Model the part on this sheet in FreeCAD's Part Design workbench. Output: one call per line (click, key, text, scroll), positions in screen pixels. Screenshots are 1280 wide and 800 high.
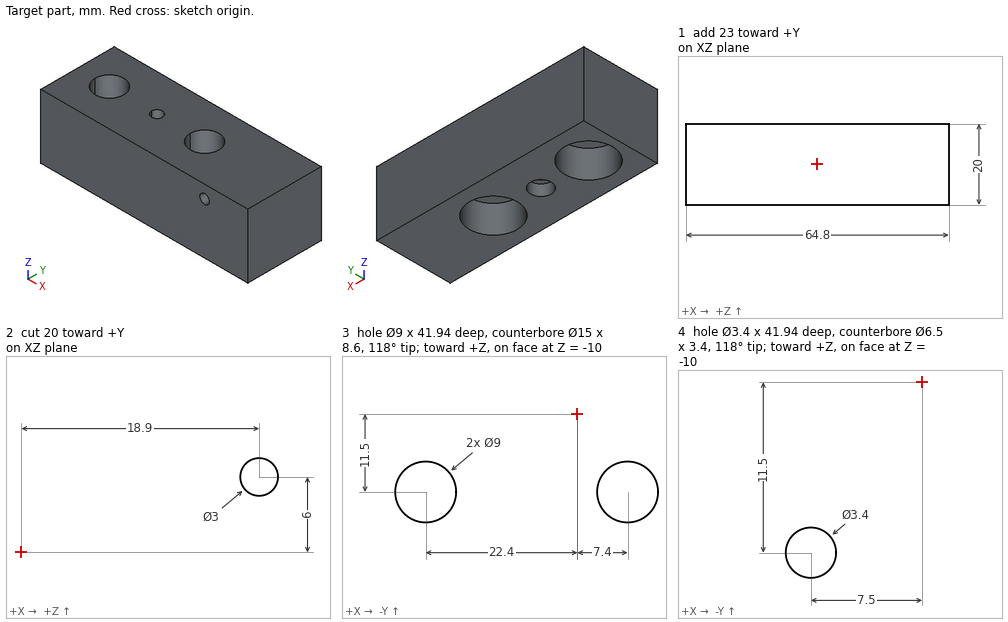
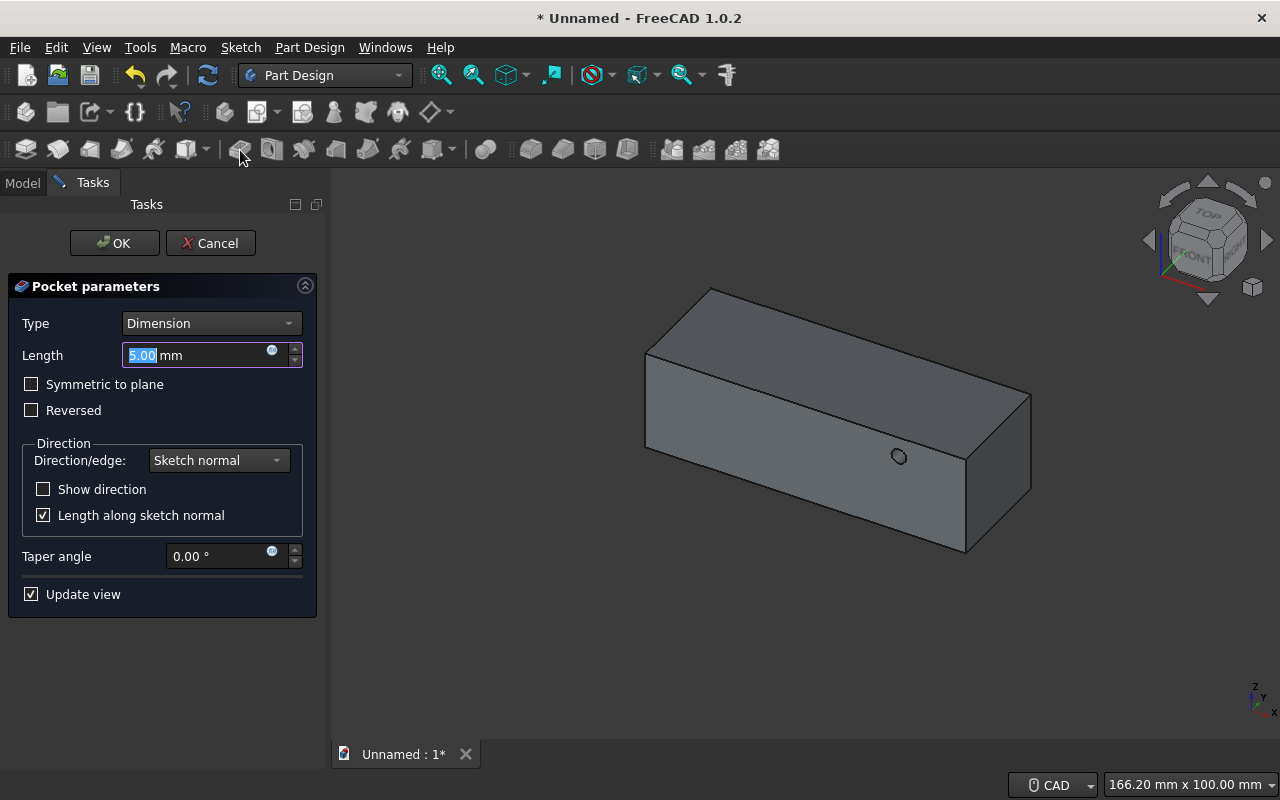
text(20)
key(Tab)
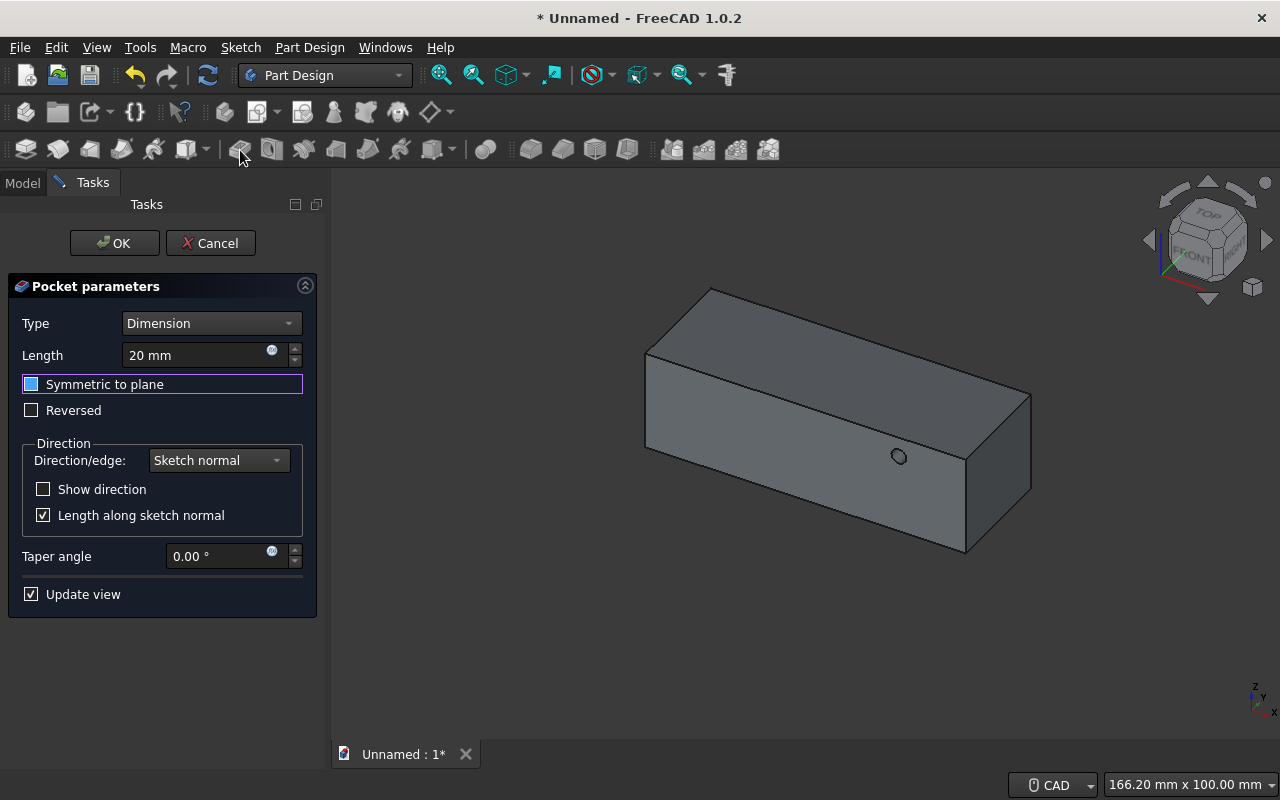
click(115, 243)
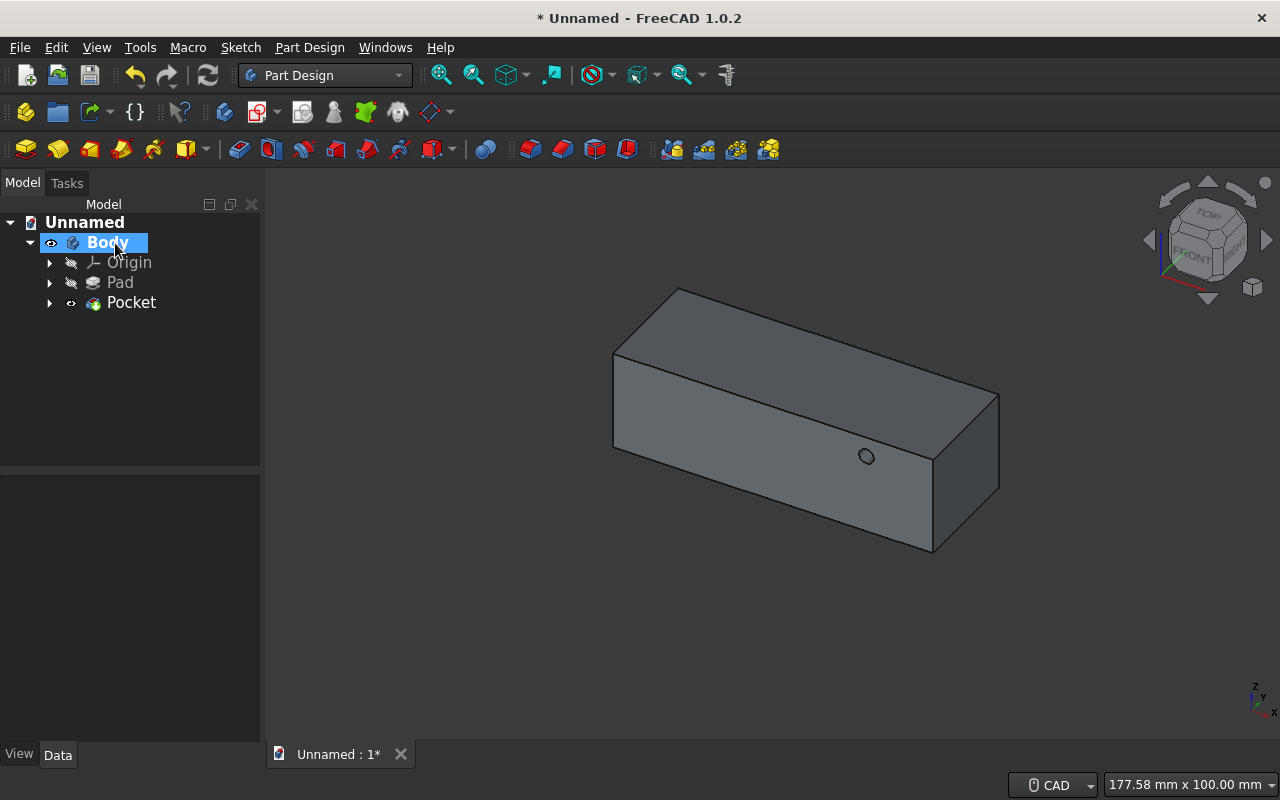
key(5)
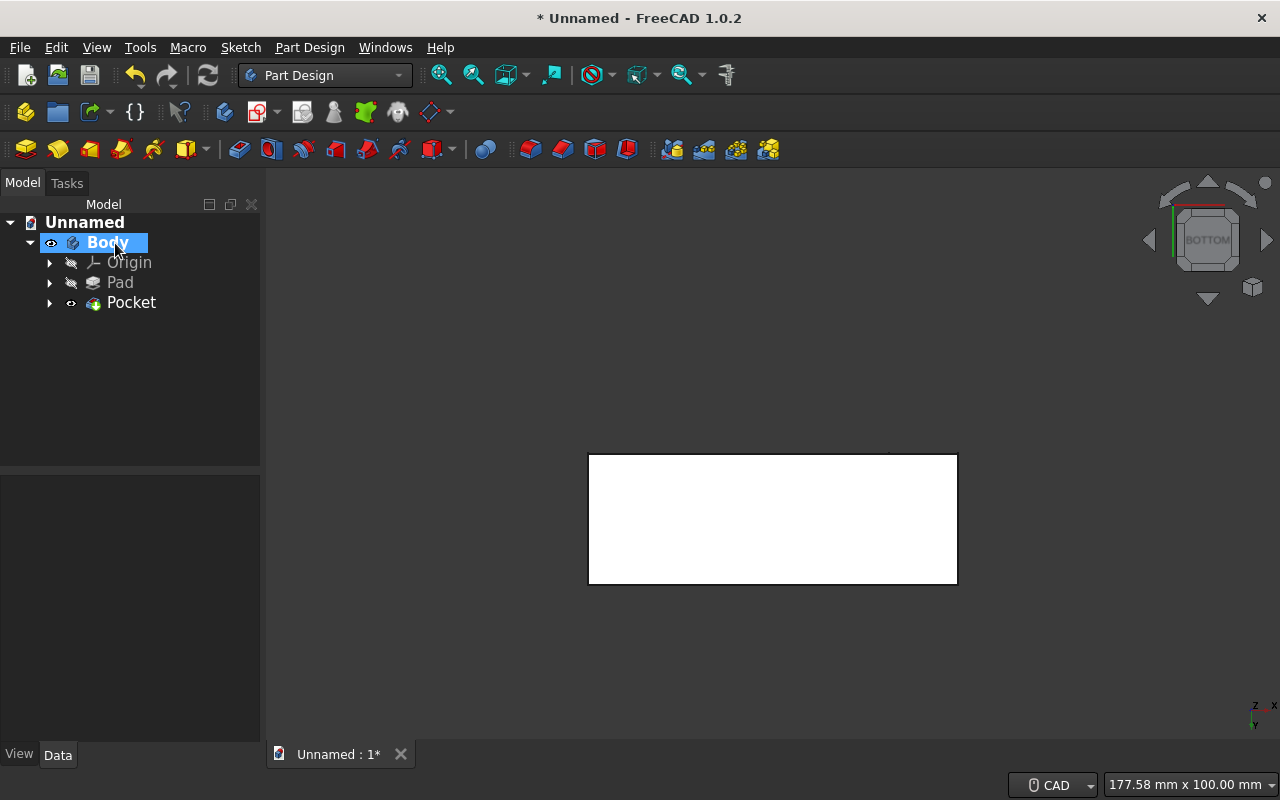
click(442, 76)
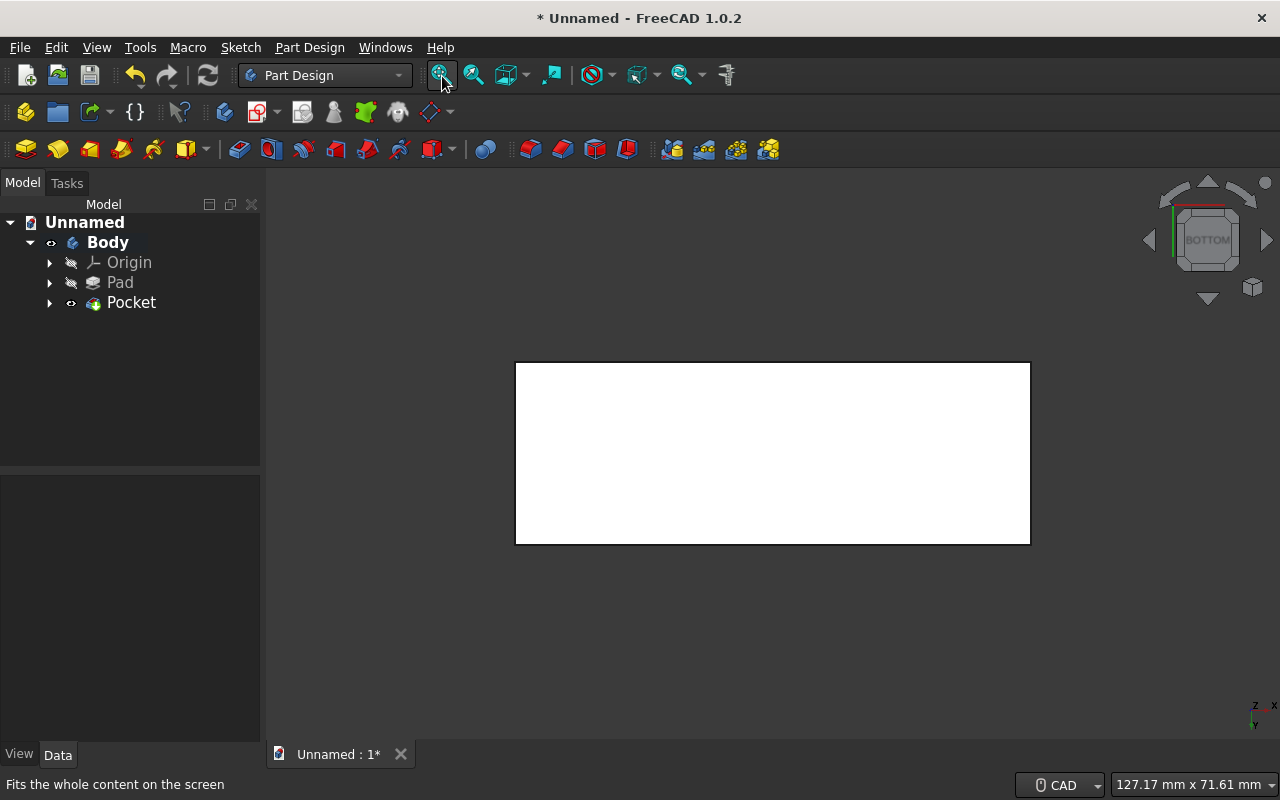
click(921, 452)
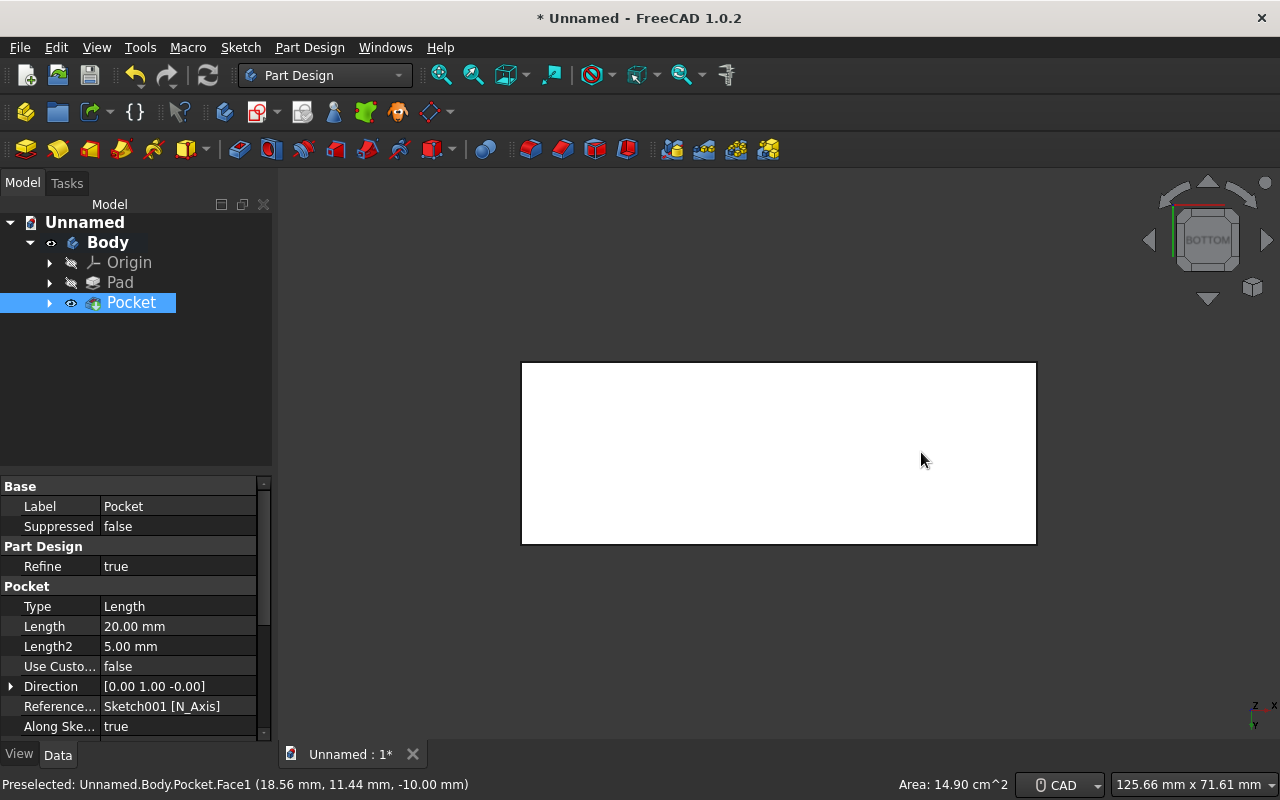
click(258, 112)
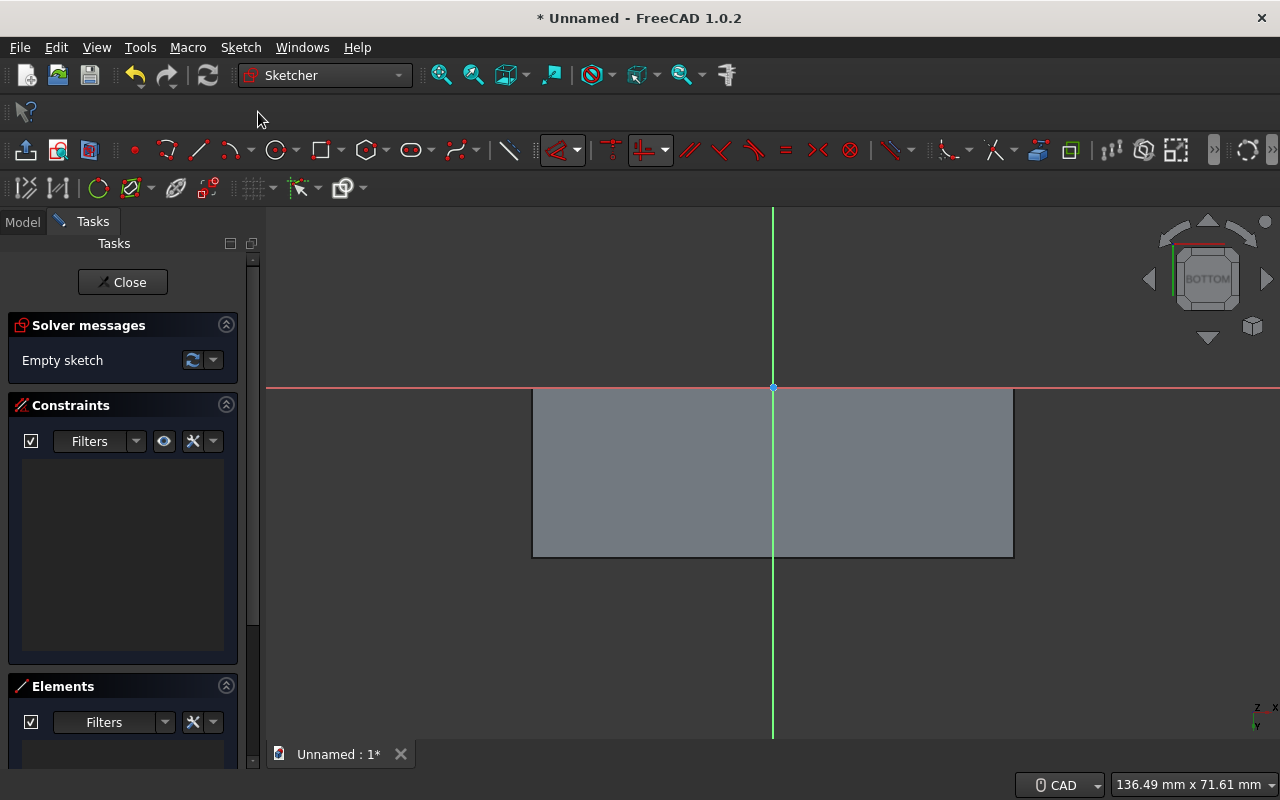
scroll(733, 415, up, 3)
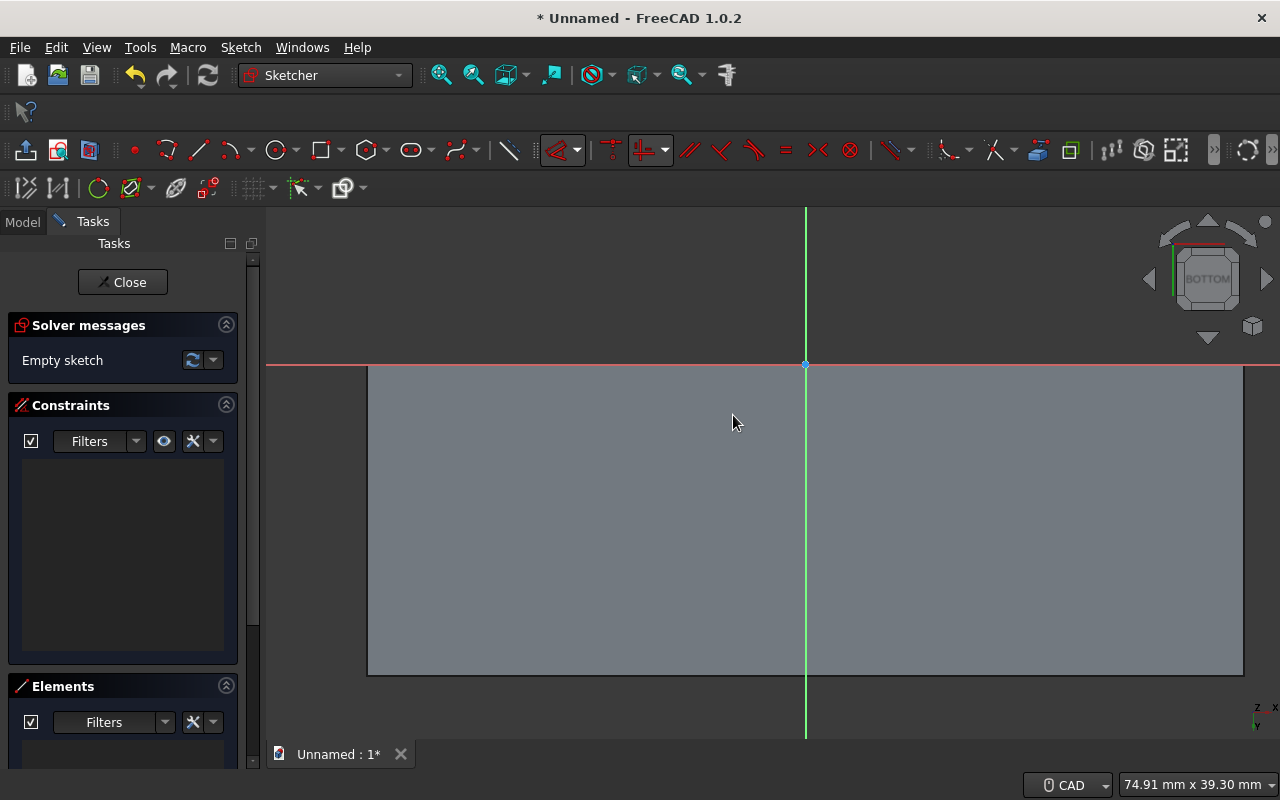
click(276, 150)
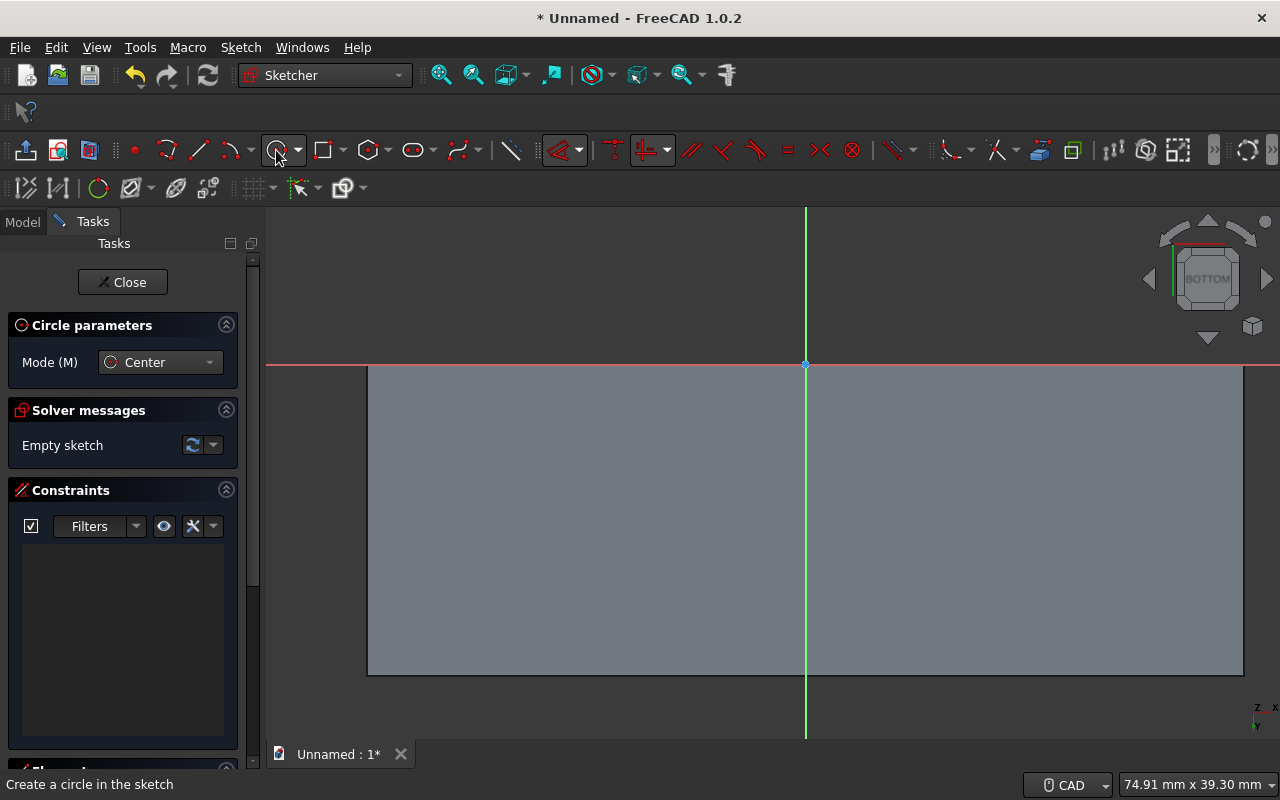
click(502, 520)
move(545, 477)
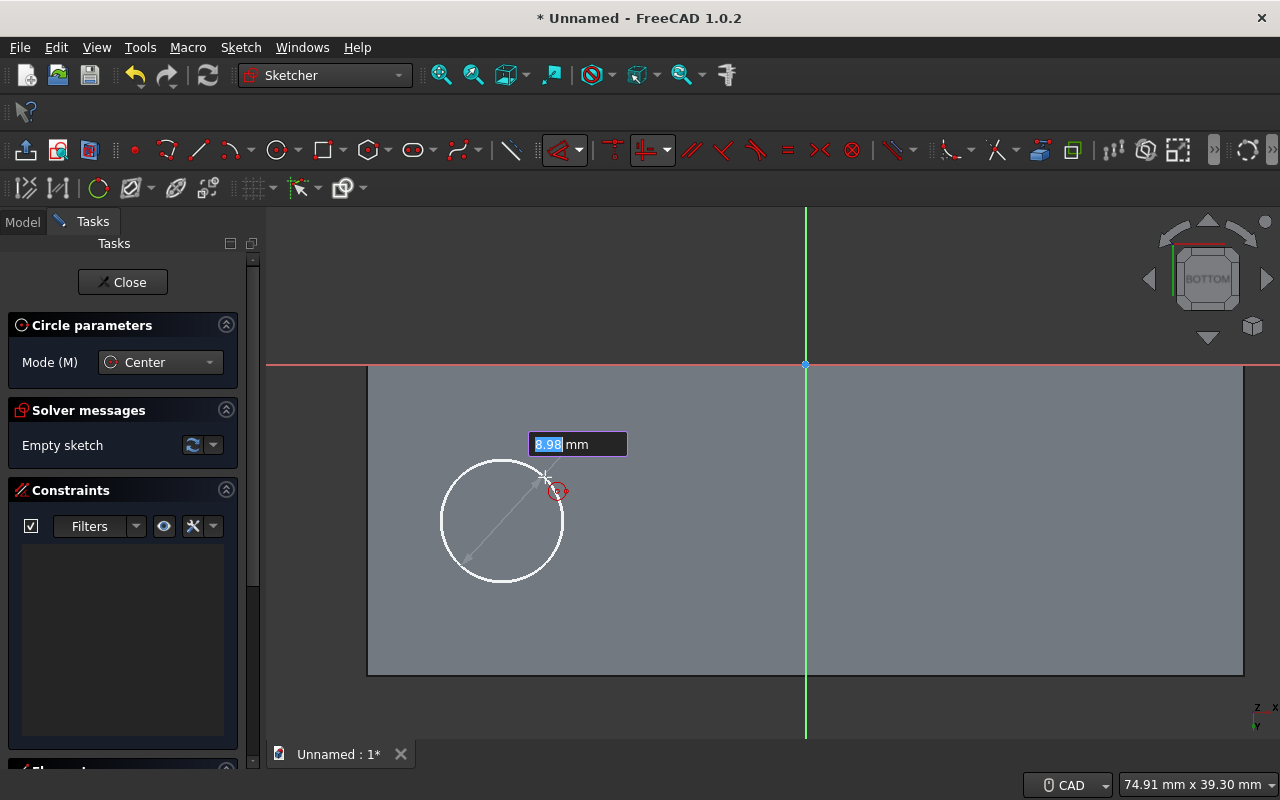
text(9)
key(Return)